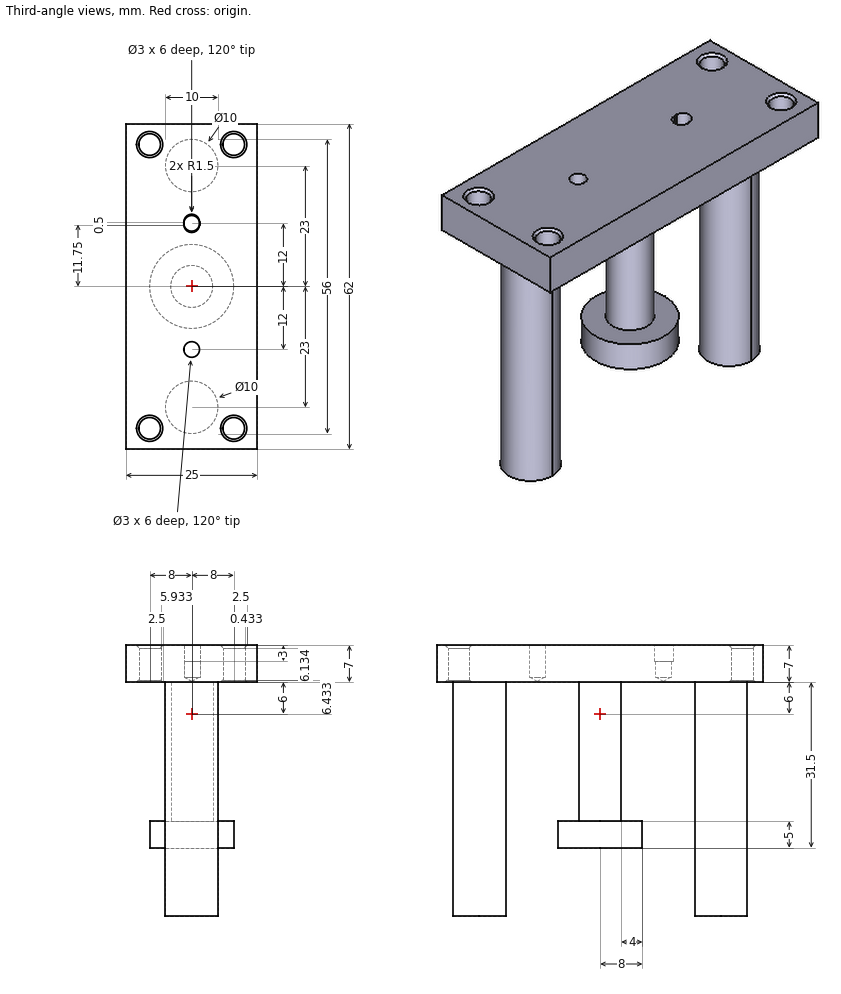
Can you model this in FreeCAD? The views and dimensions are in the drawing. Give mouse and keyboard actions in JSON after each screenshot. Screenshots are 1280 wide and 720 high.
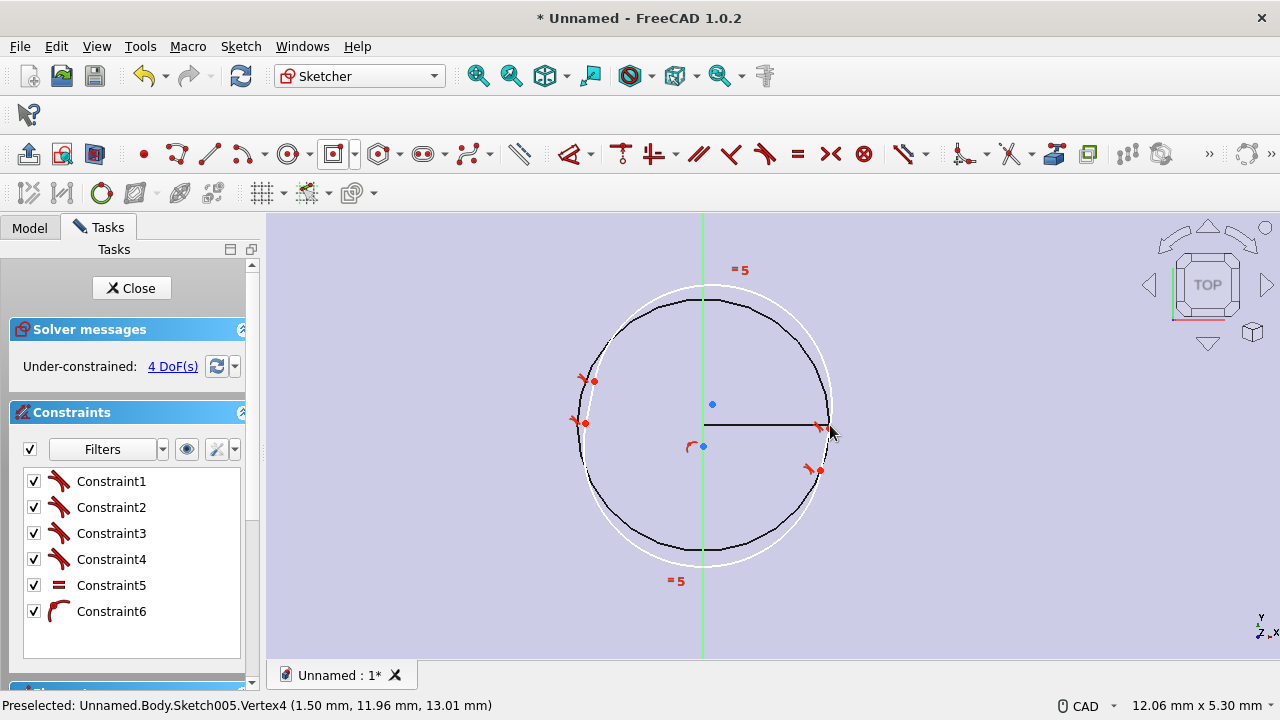
{"action": "left_click", "coordinate": [568, 154]}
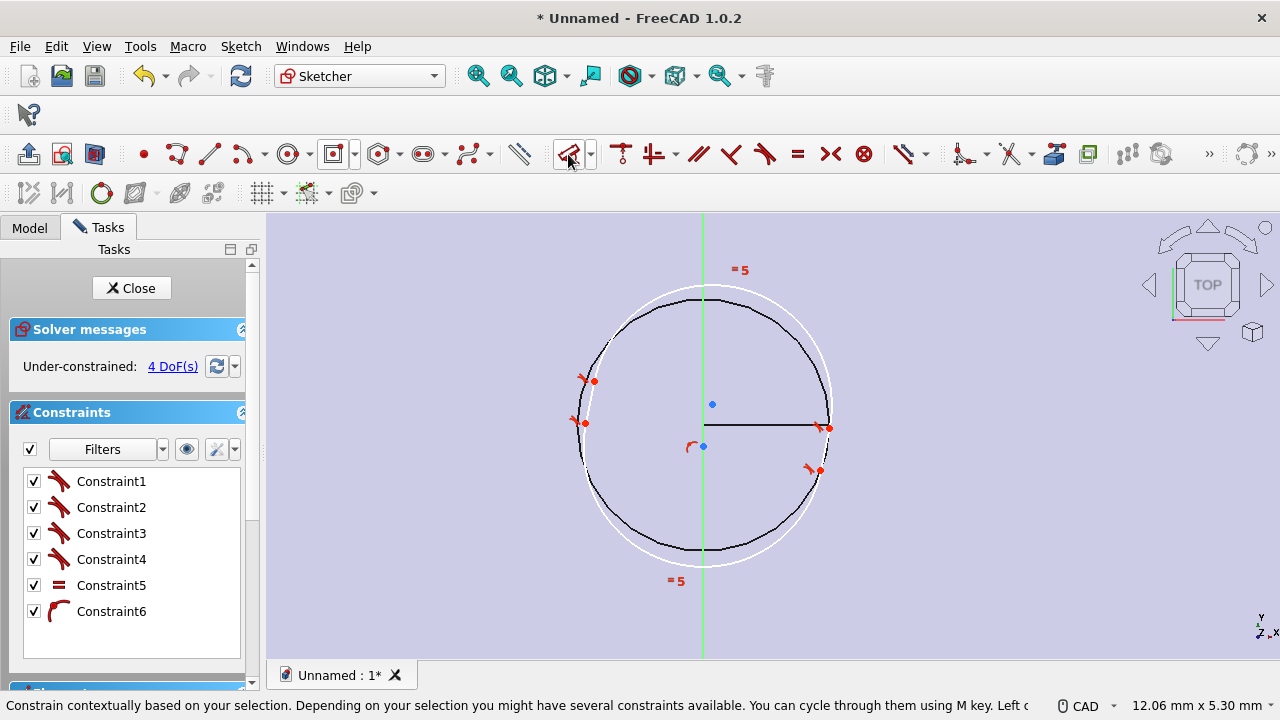
{"action": "left_click", "coordinate": [615, 528]}
{"action": "left_click", "coordinate": [591, 550]}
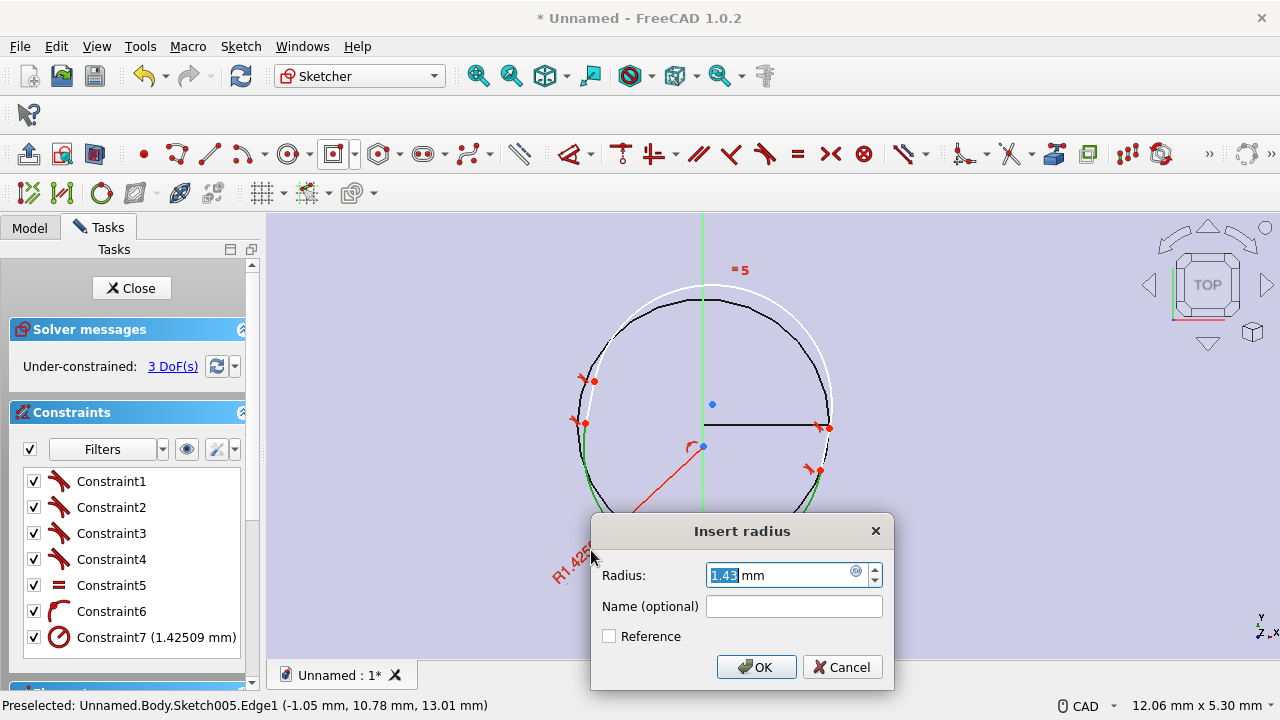
{"action": "type", "text": "1.5"}
{"action": "key", "text": "Return"}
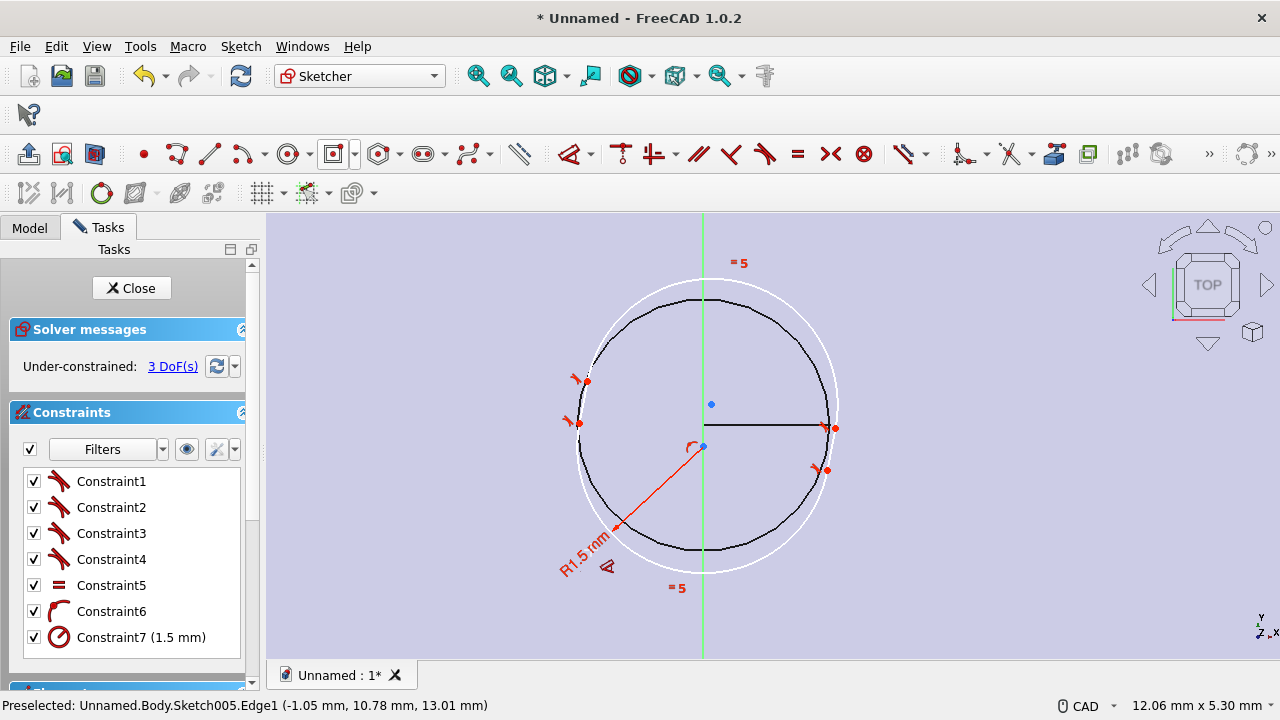
{"action": "left_click", "coordinate": [582, 410]}
{"action": "left_click", "coordinate": [546, 402]}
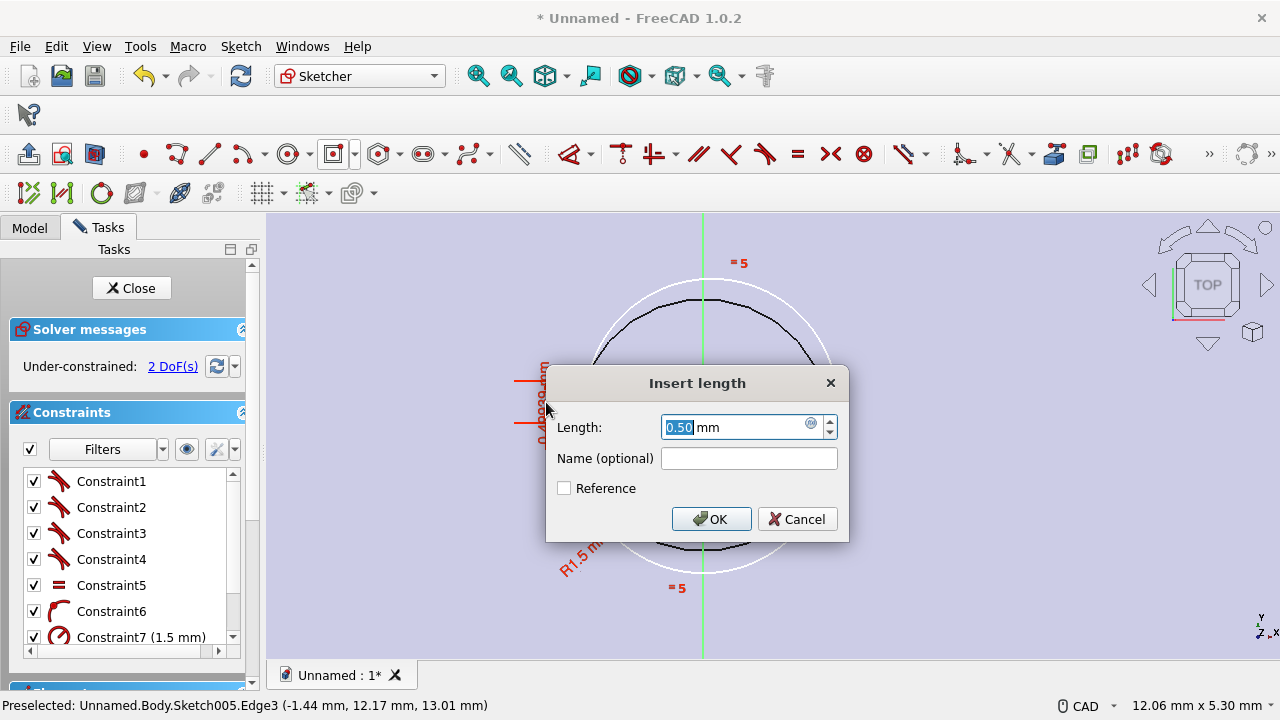
{"action": "type", "text": "0.5"}
{"action": "key", "text": "Return"}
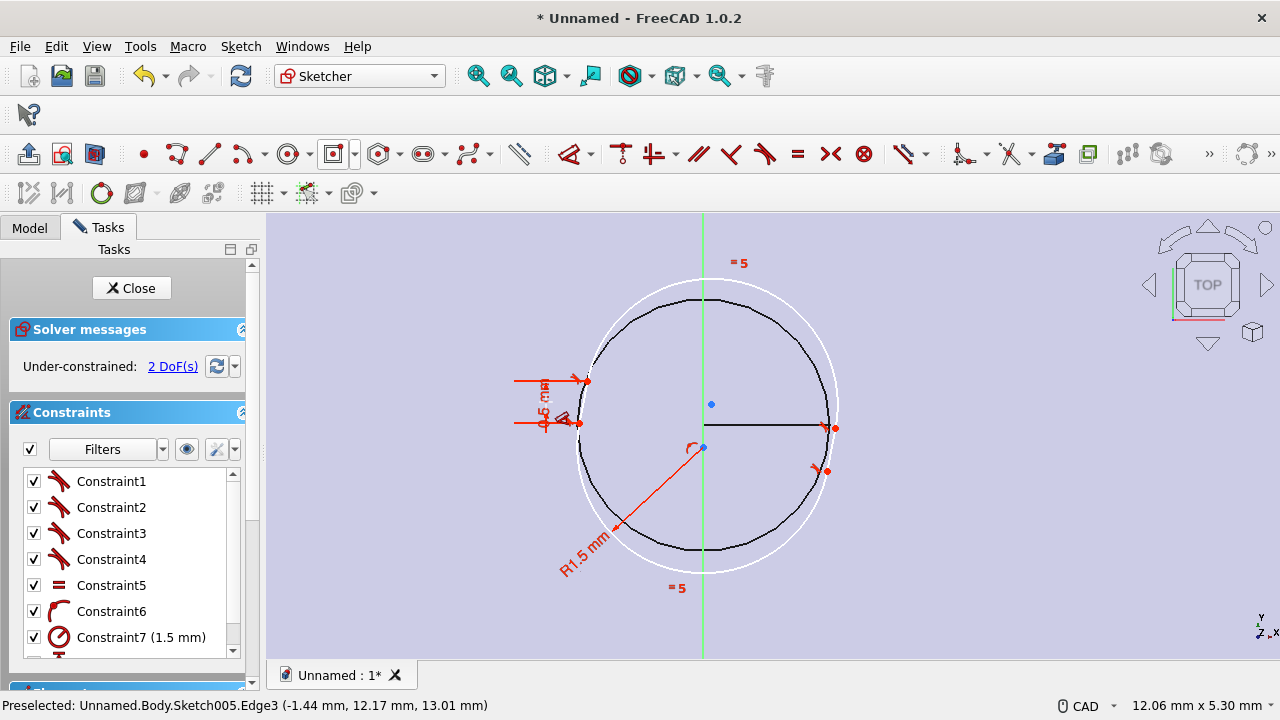
{"action": "left_click", "coordinate": [580, 423]}
{"action": "left_click", "coordinate": [546, 527]}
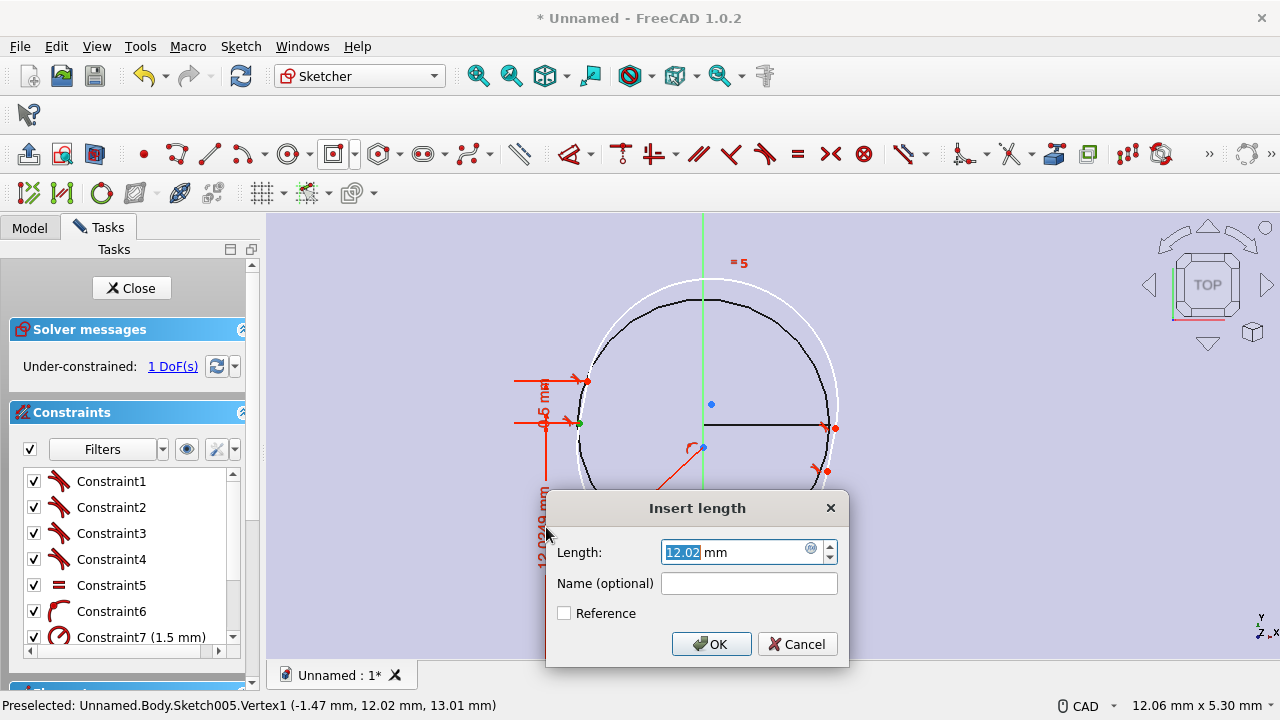
{"action": "type", "text": "11.75"}
{"action": "key", "text": "Return"}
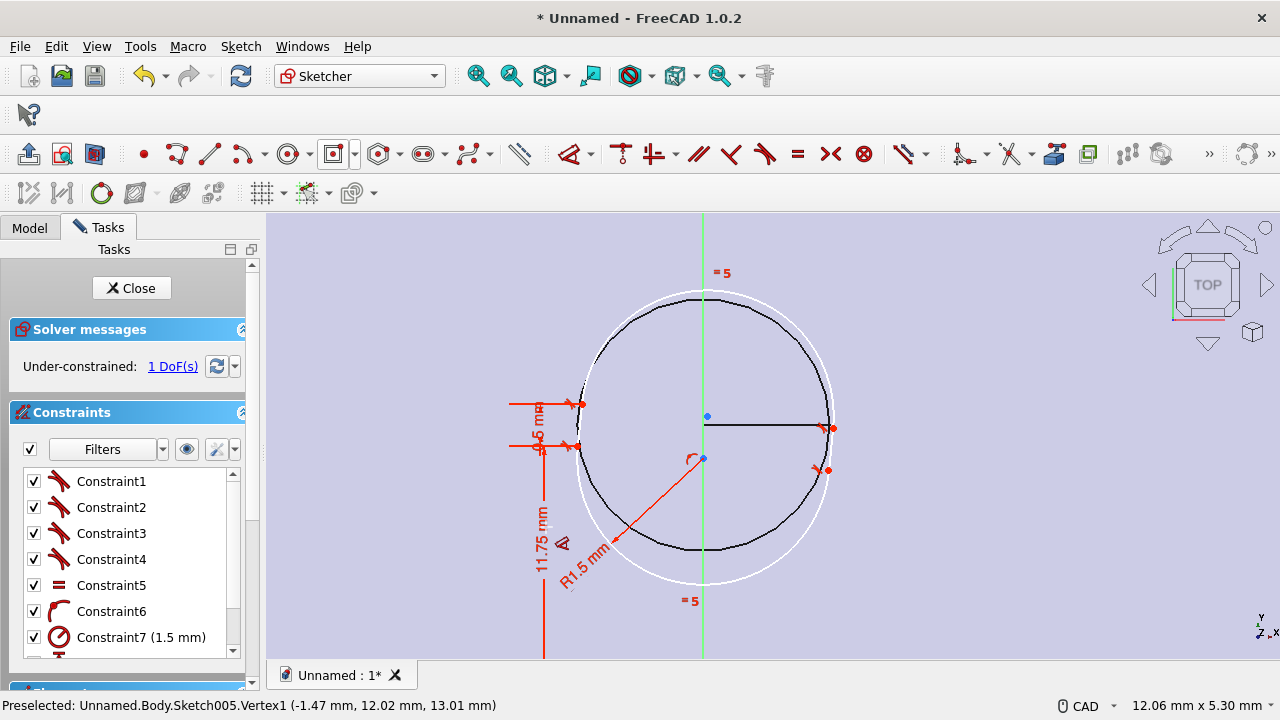
{"action": "left_click", "coordinate": [829, 471]}
{"action": "left_click", "coordinate": [863, 551]}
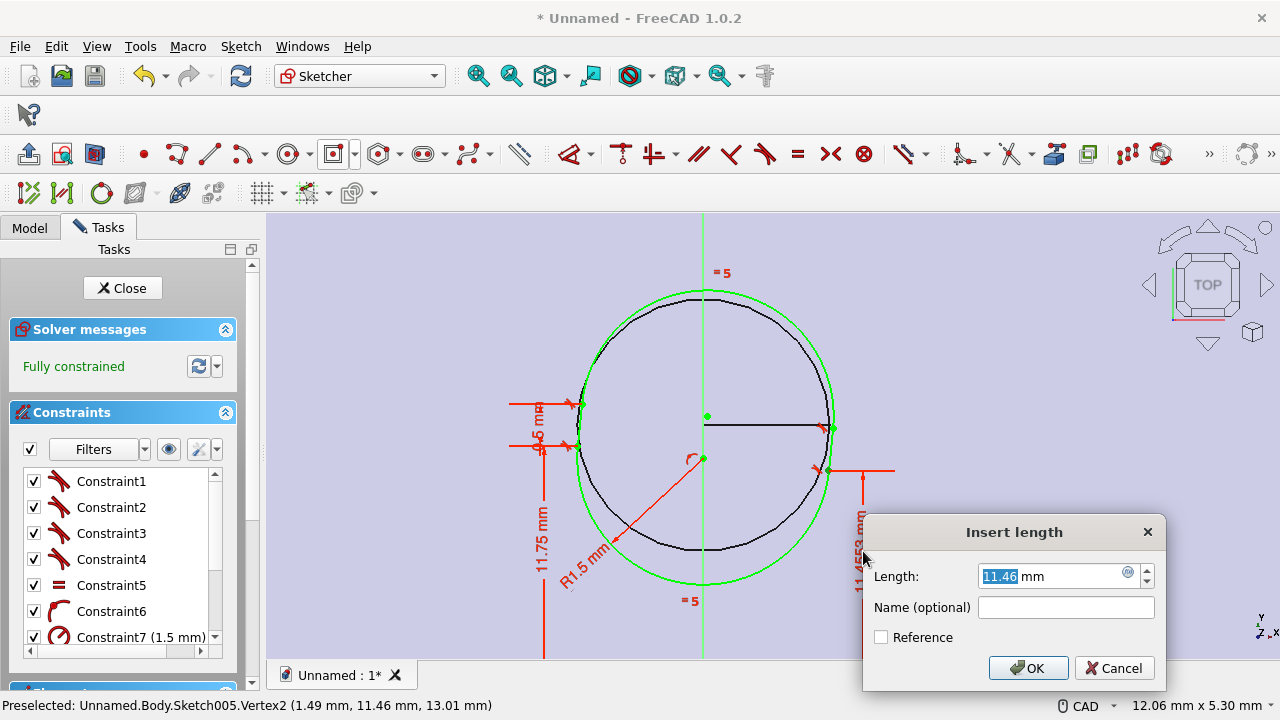
{"action": "type", "text": "11.75"}
{"action": "key", "text": "Return"}
{"action": "key", "text": "Escape"}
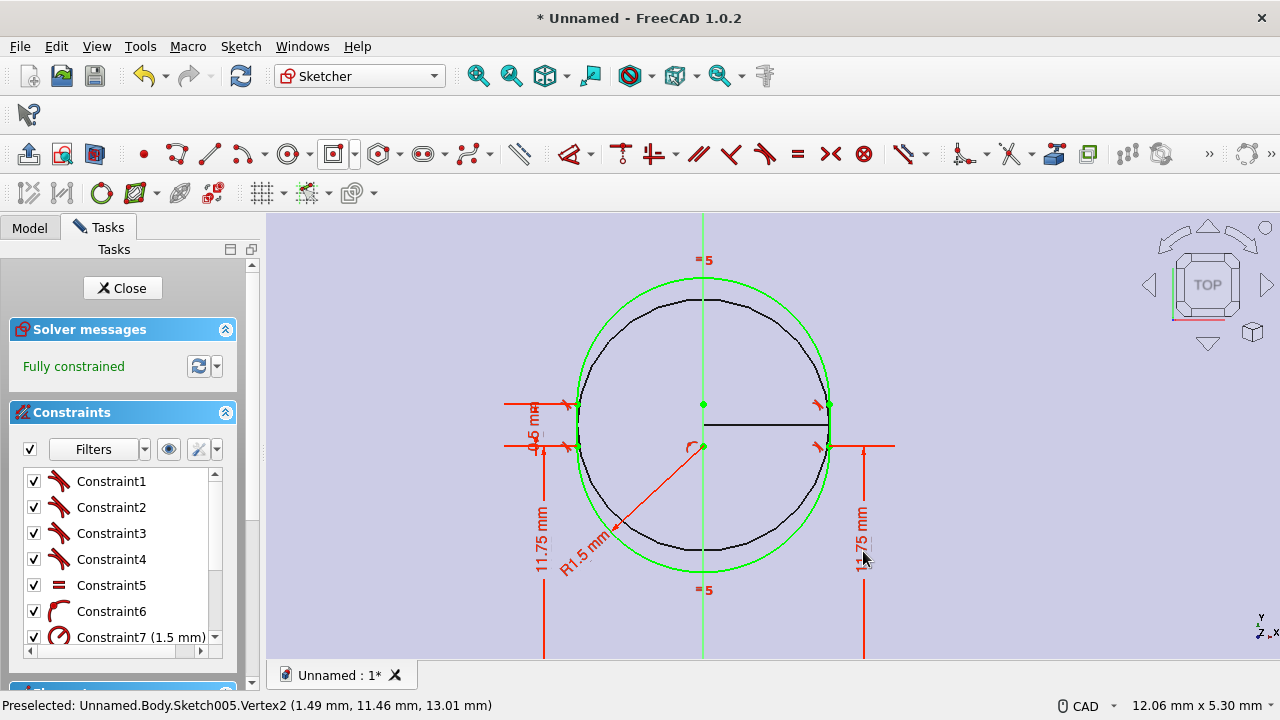
{"action": "left_click", "coordinate": [123, 288]}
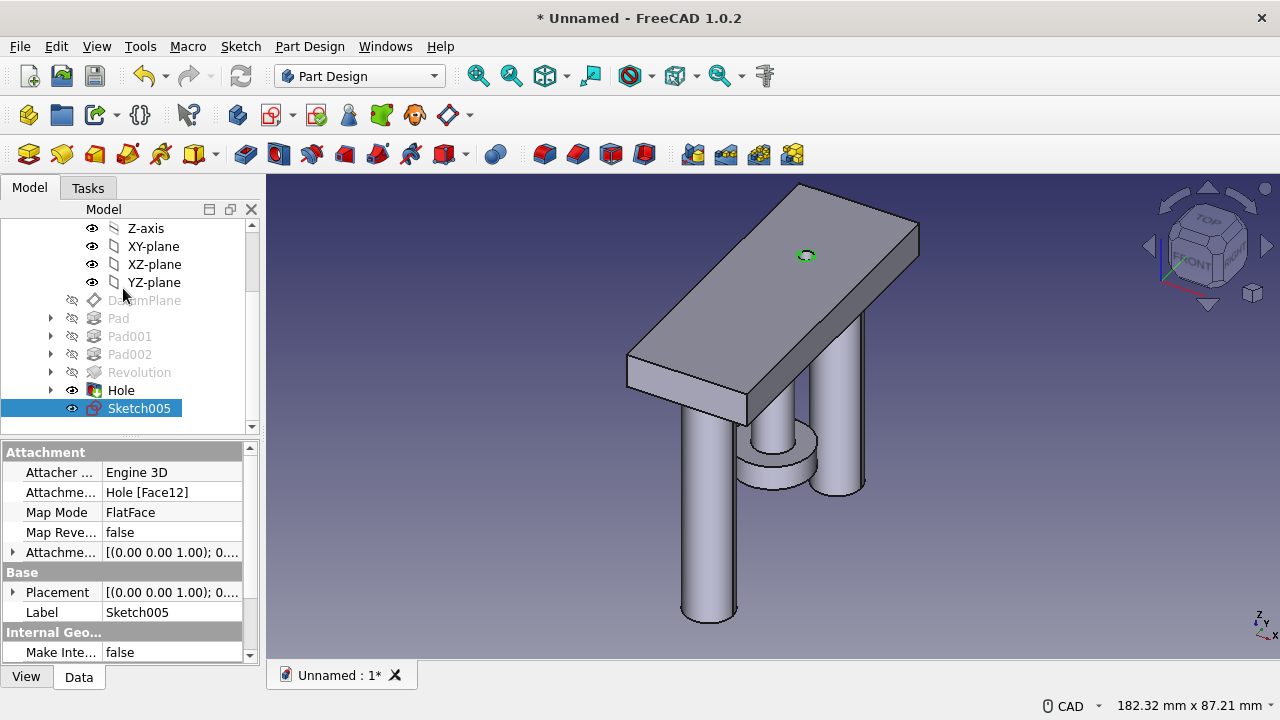
{"action": "left_click", "coordinate": [246, 154]}